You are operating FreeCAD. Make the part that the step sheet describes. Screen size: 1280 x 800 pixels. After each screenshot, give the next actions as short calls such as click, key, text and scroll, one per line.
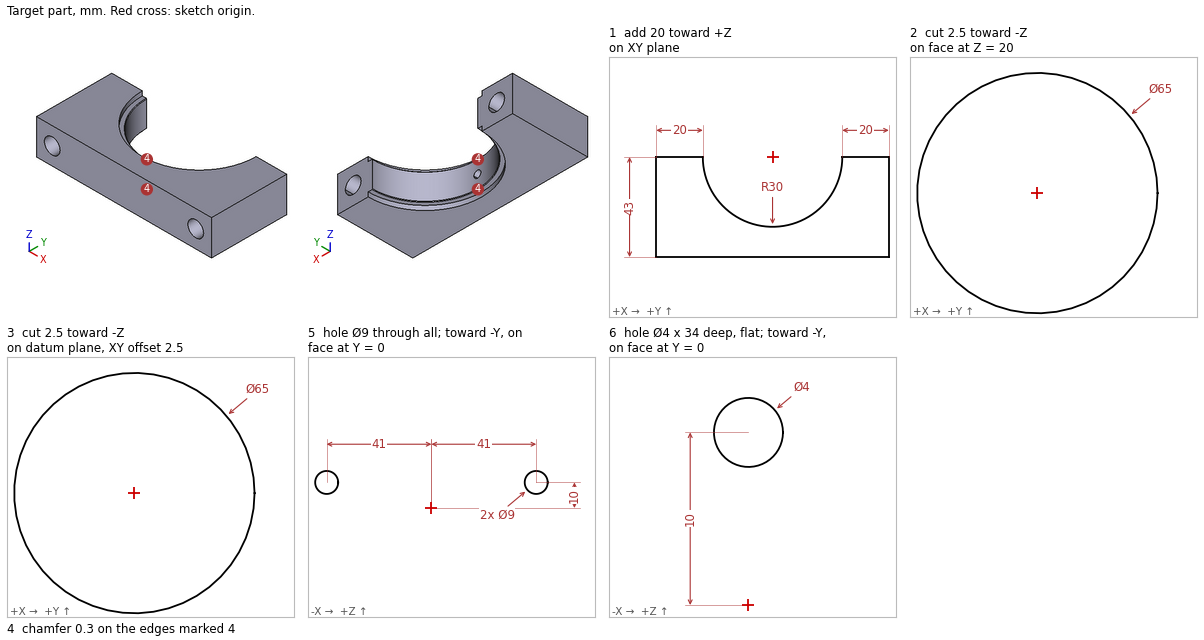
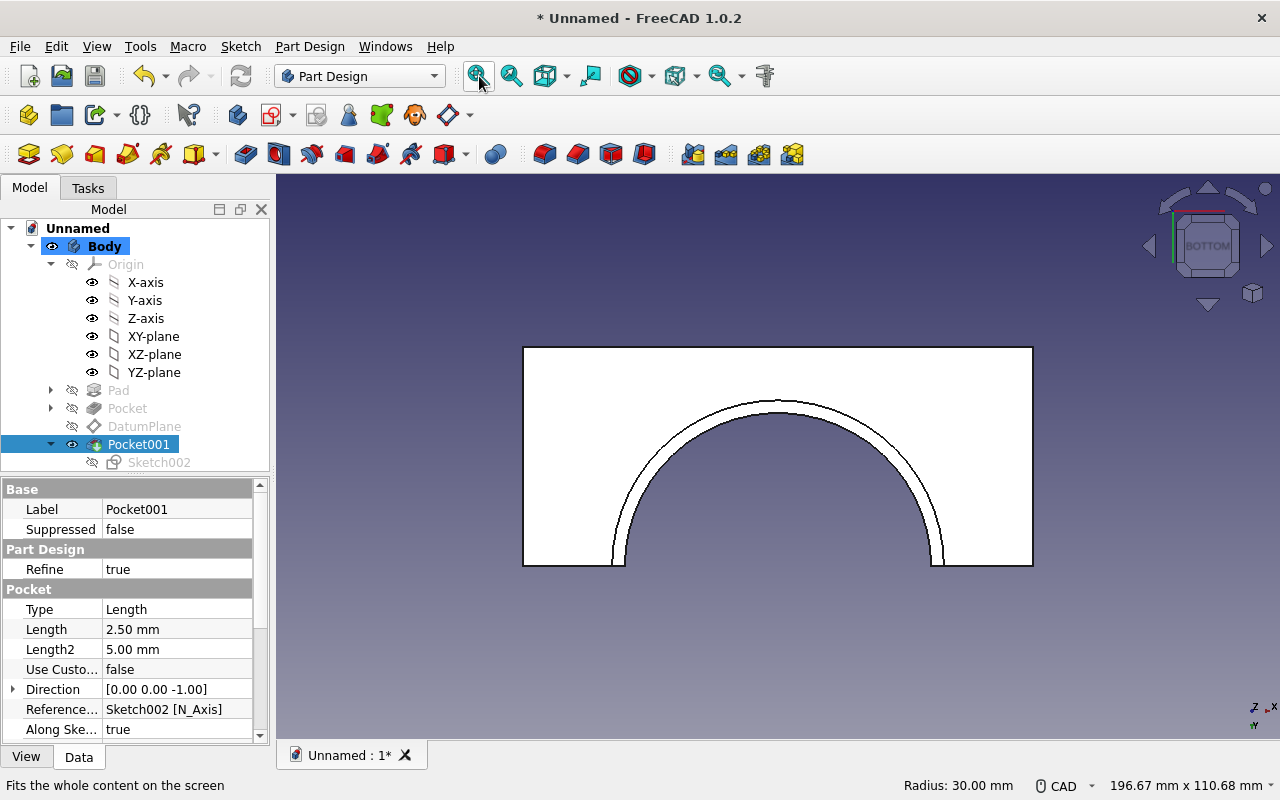
click(778, 412, ctrl)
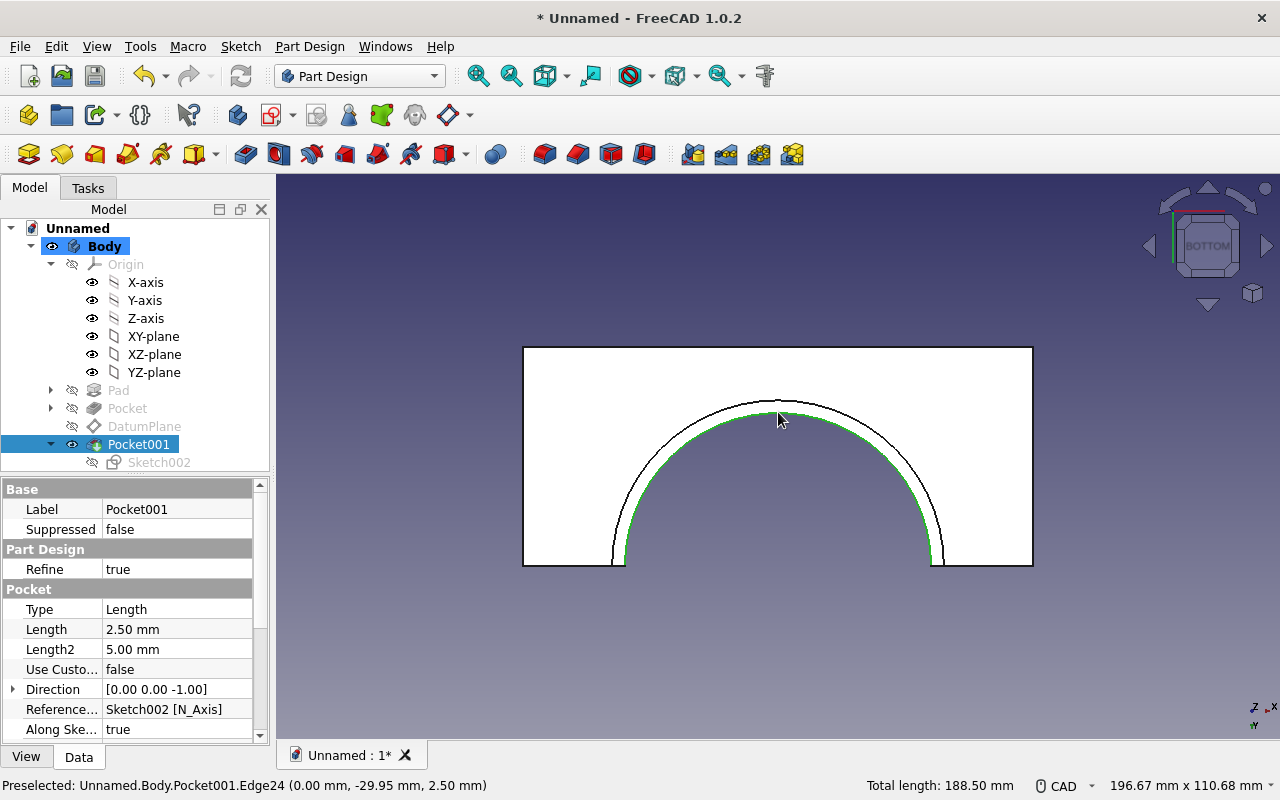
click(578, 154)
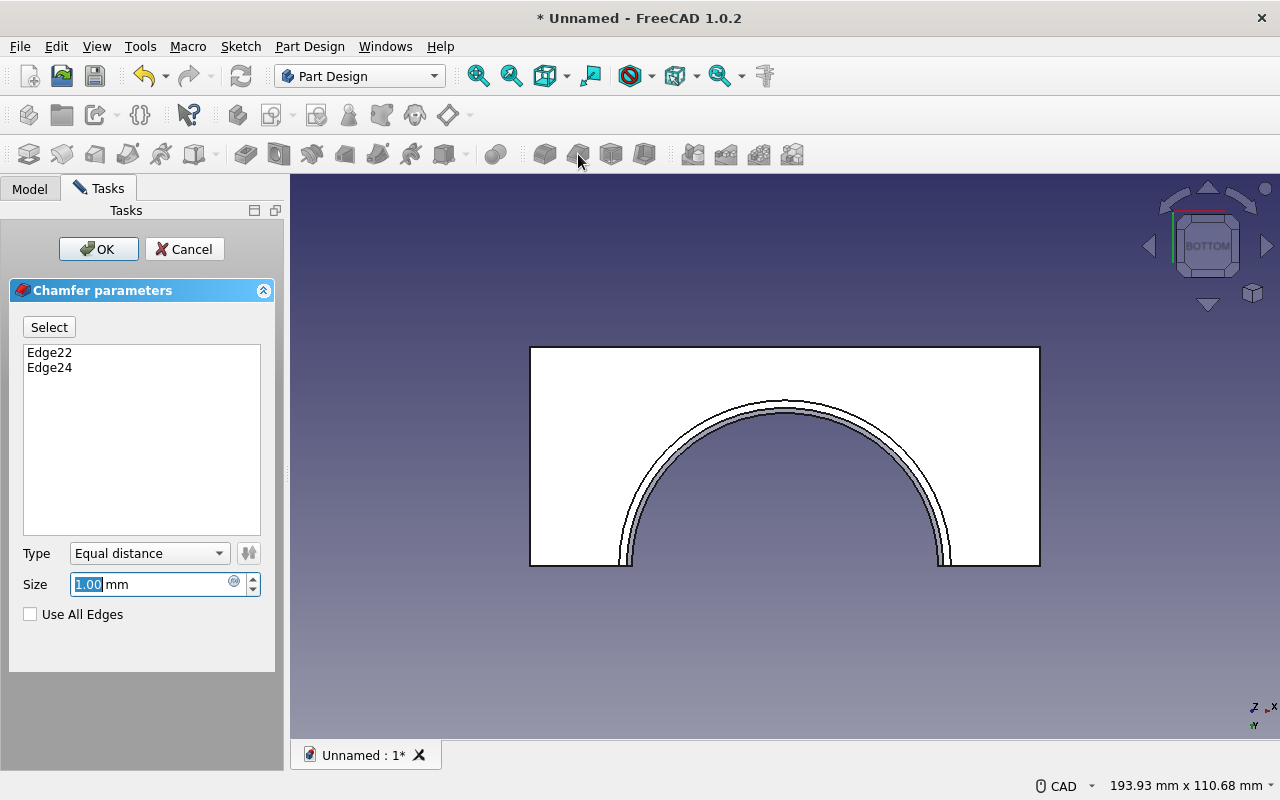
text(0.3)
key(Tab)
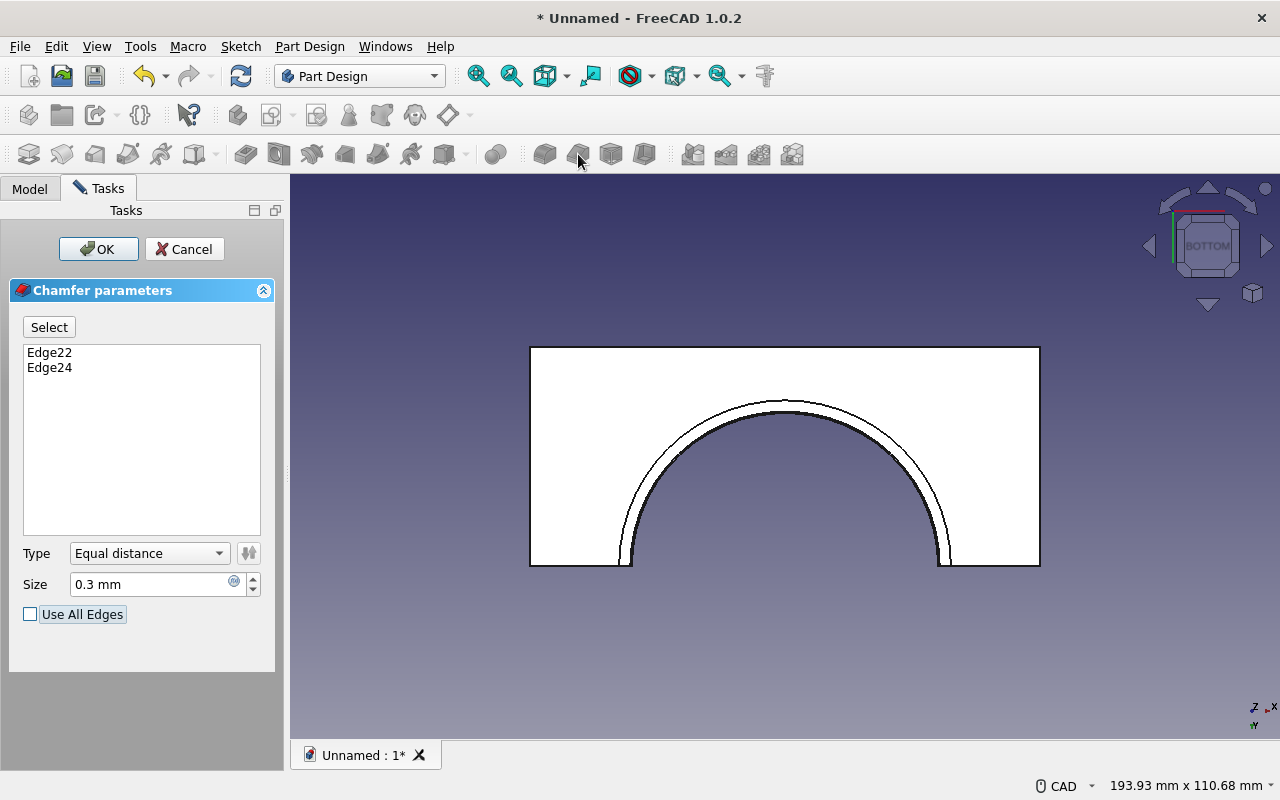
click(99, 249)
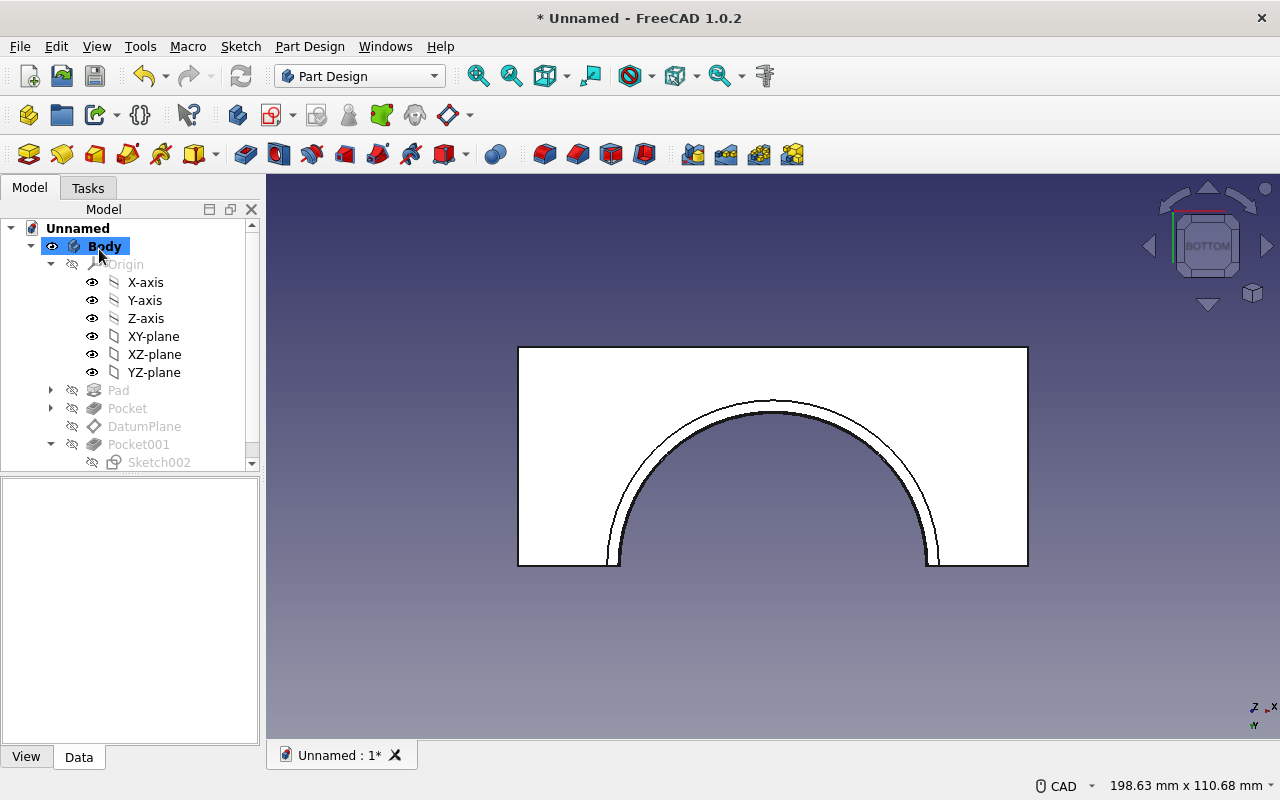
key(4)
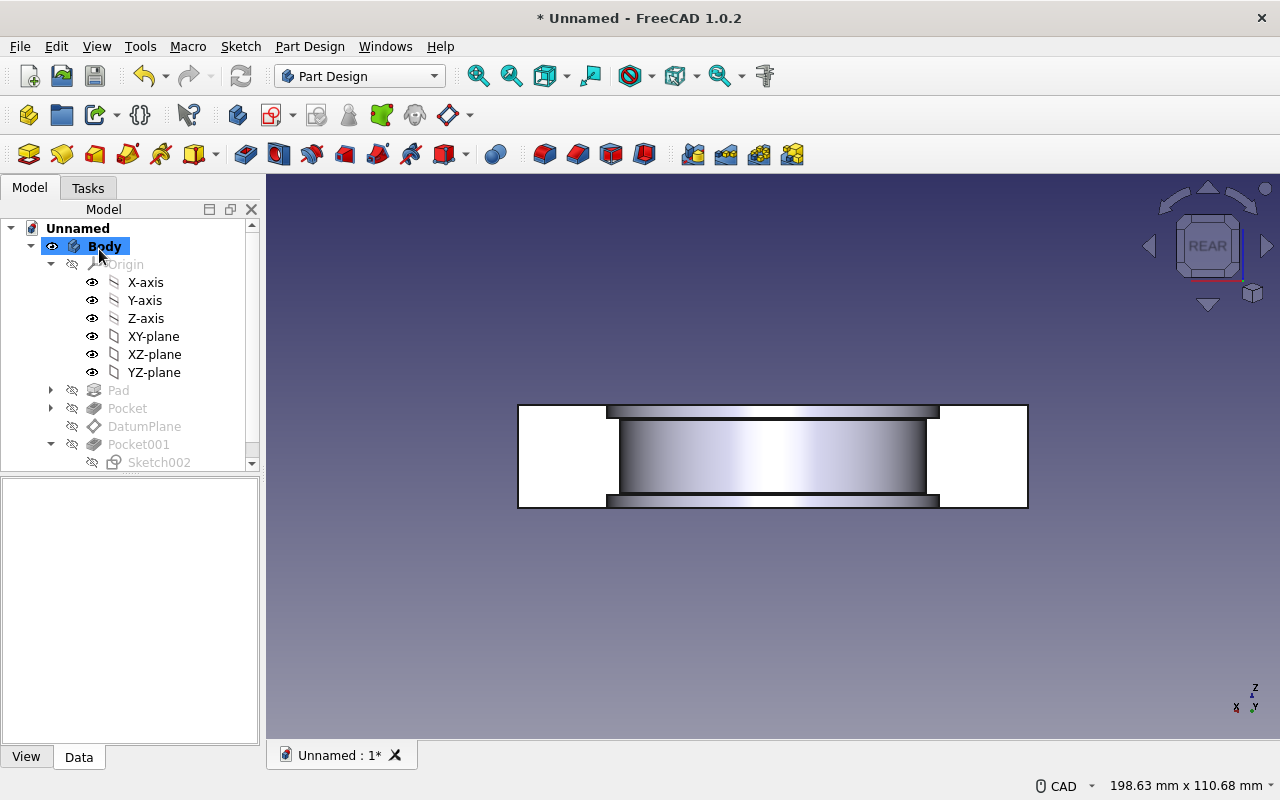
click(569, 455)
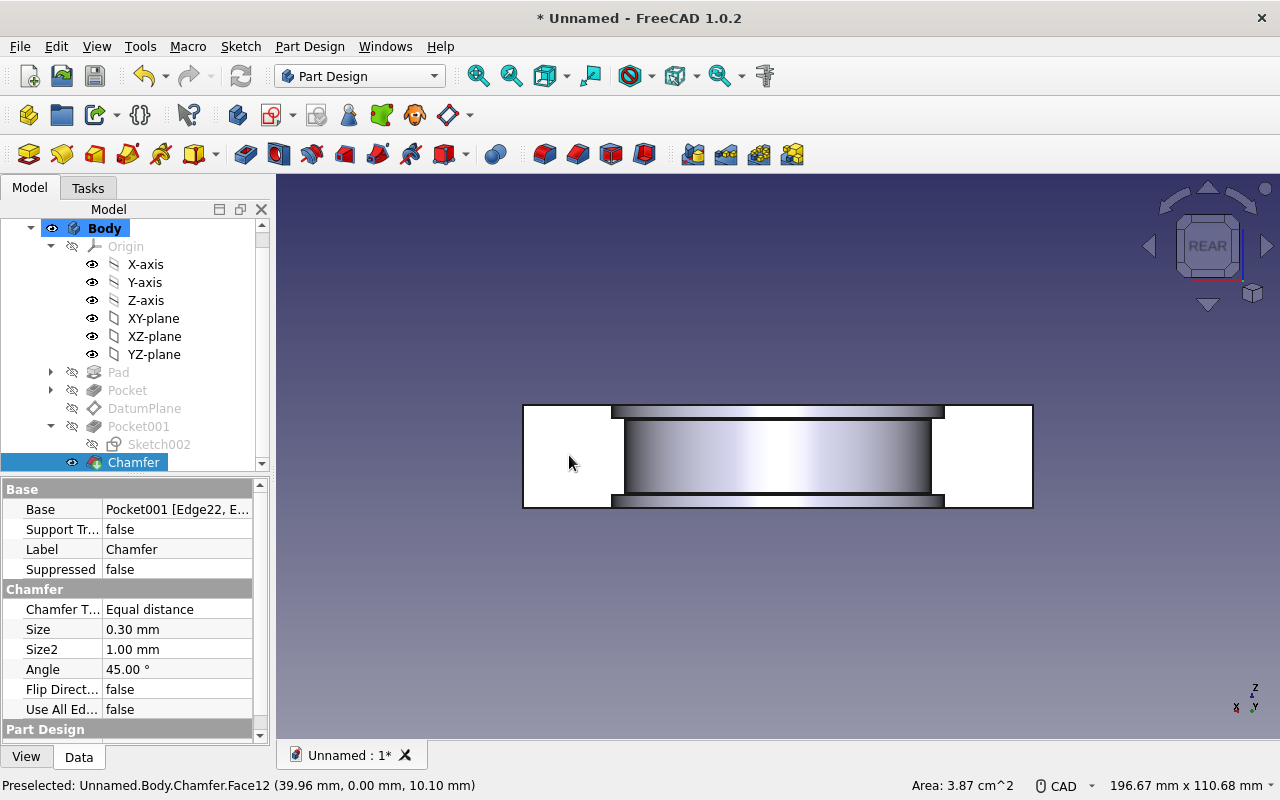
click(270, 116)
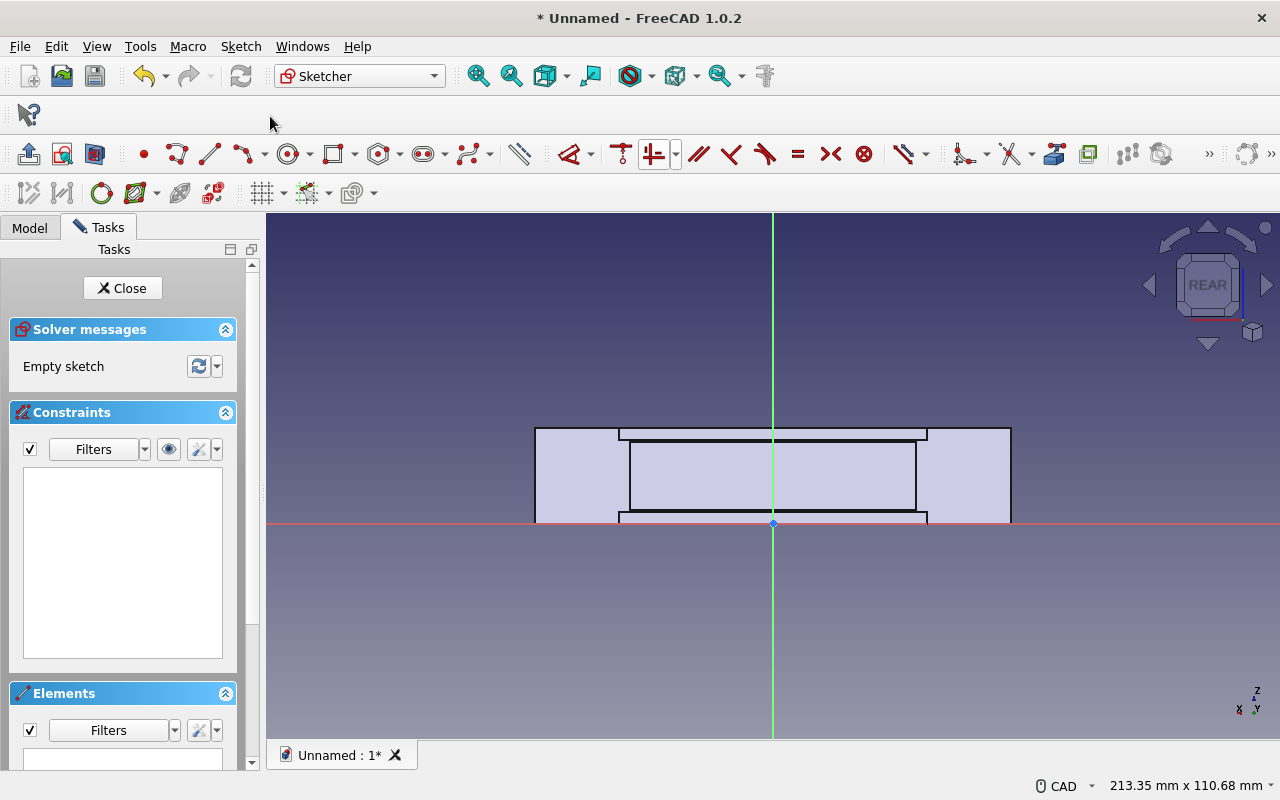
key(g)
key(c)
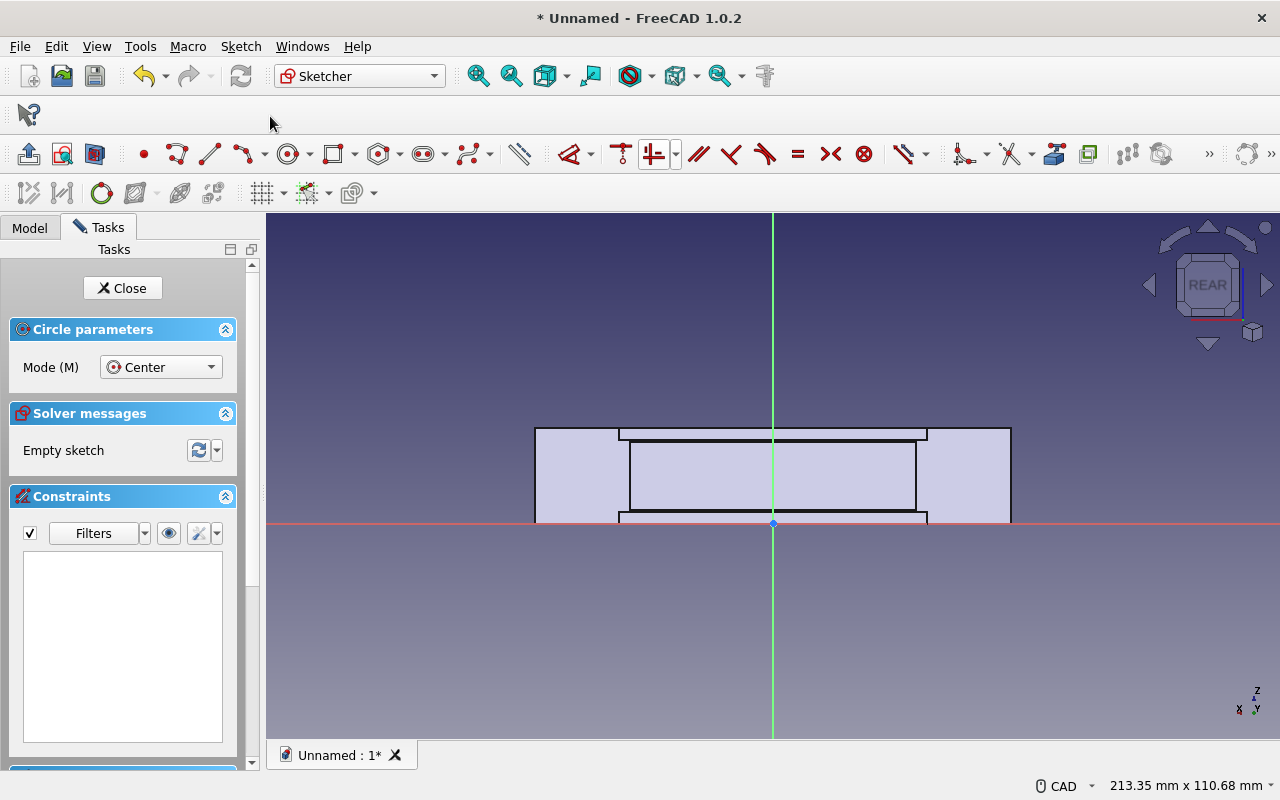
click(968, 476)
click(983, 461)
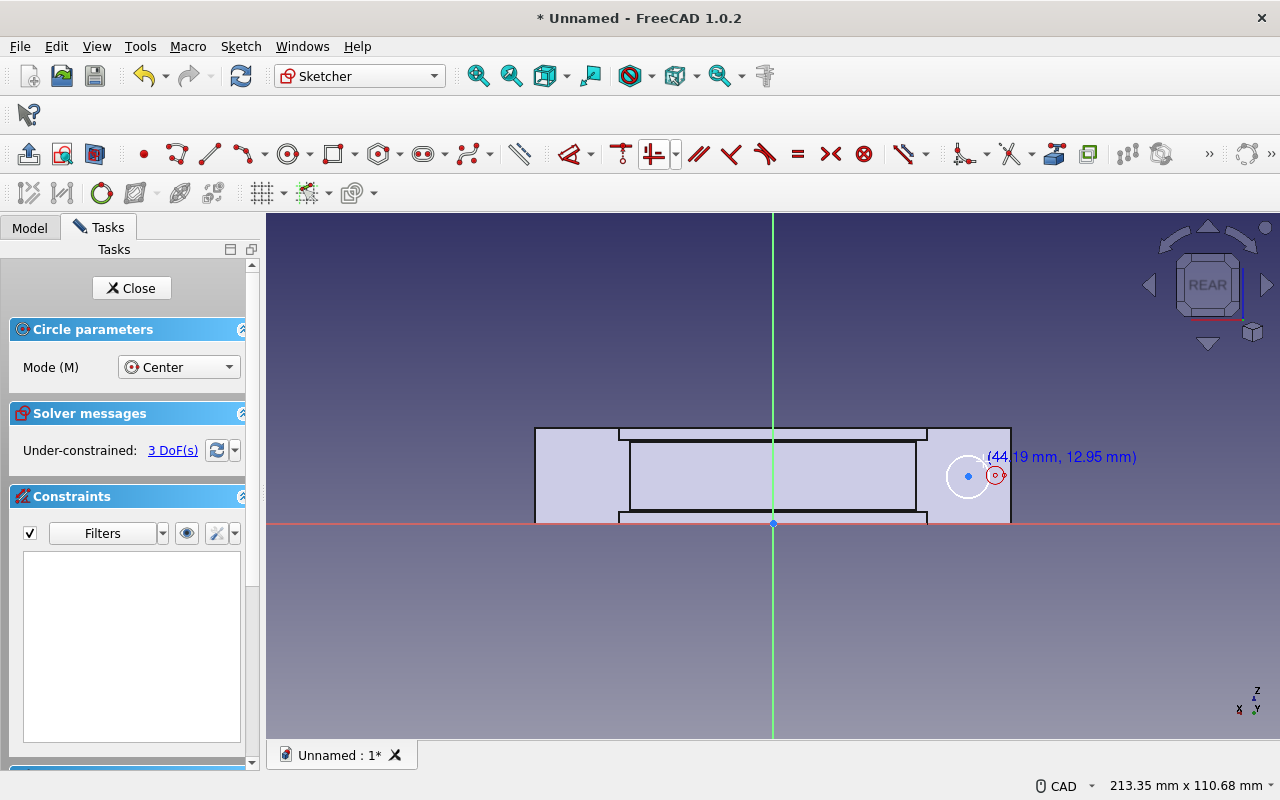
click(578, 476)
click(593, 461)
key(Escape)